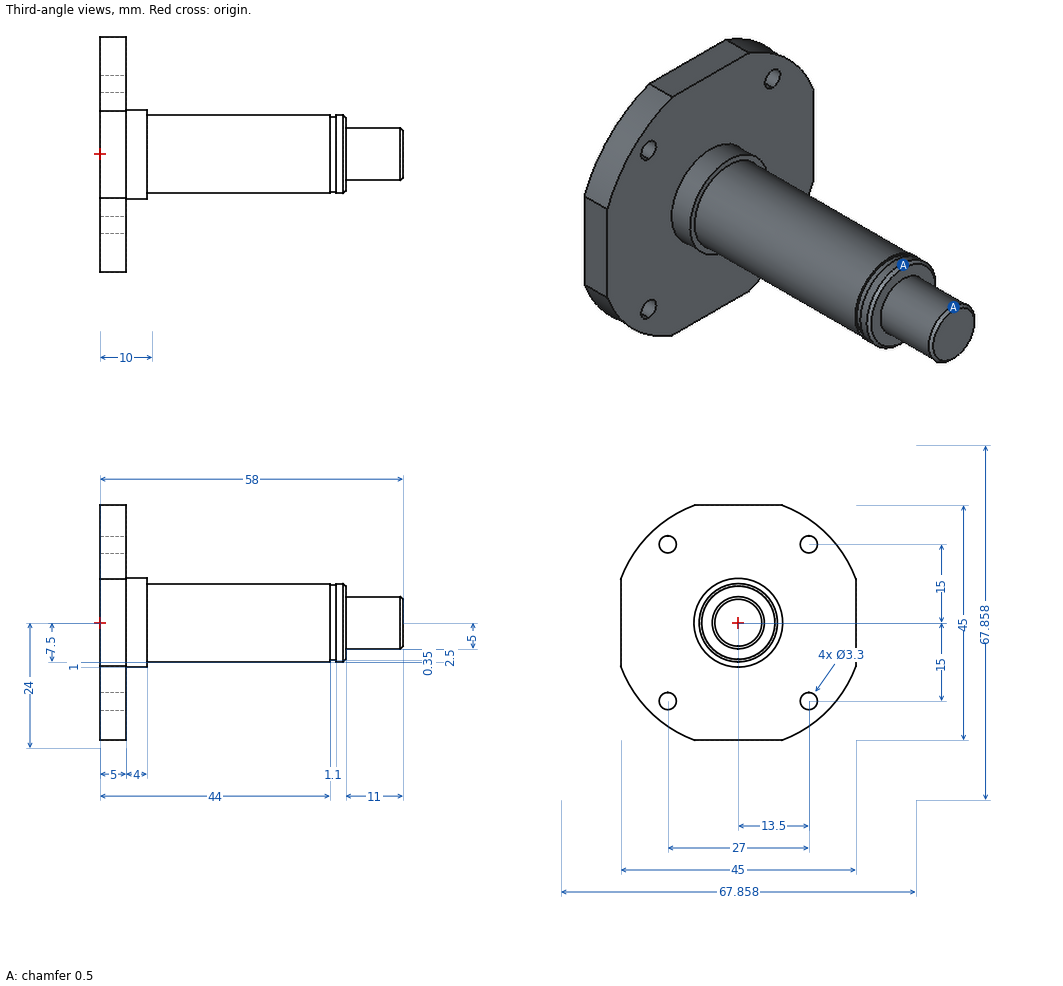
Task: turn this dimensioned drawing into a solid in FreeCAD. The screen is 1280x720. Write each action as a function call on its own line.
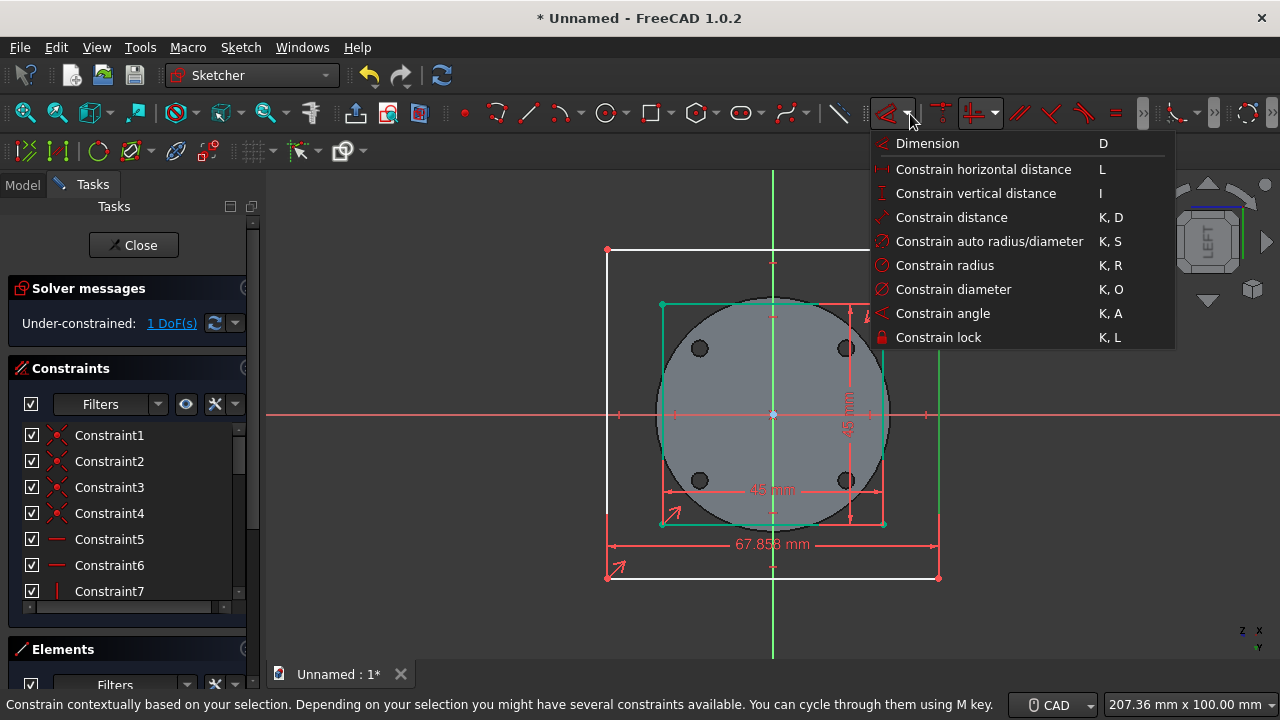
click(1023, 193)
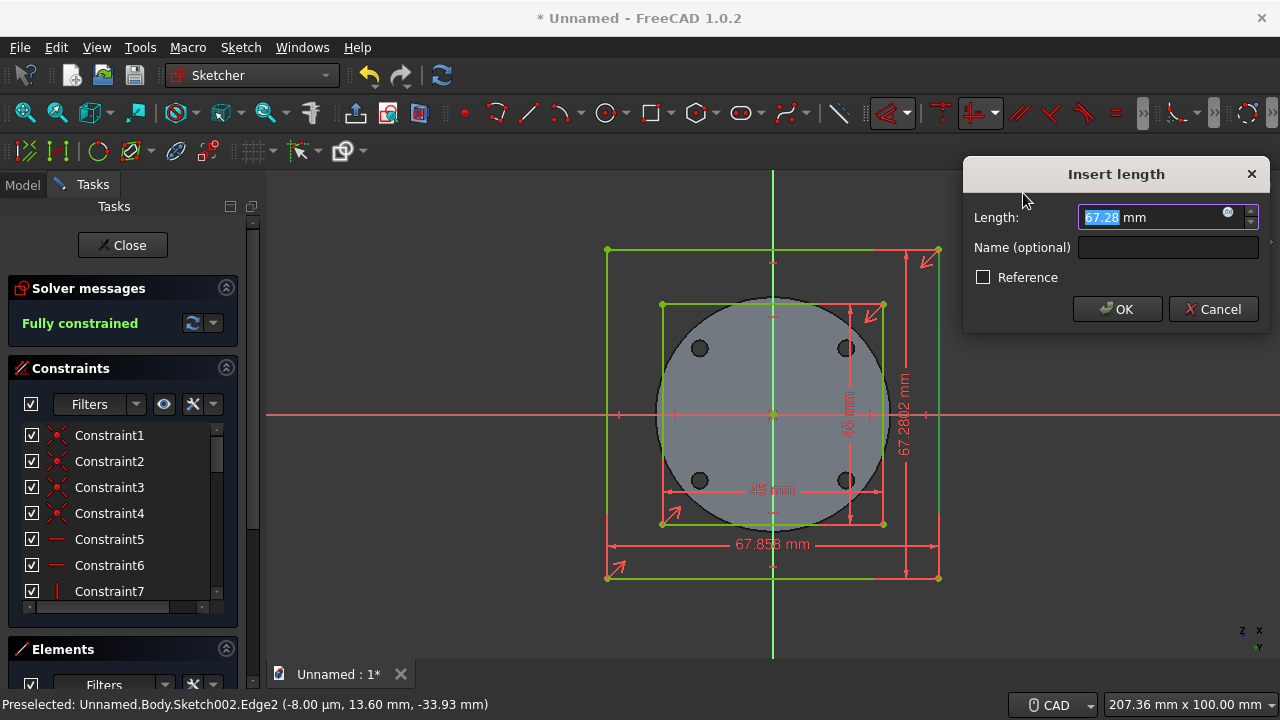
text(67.858)
key(Return)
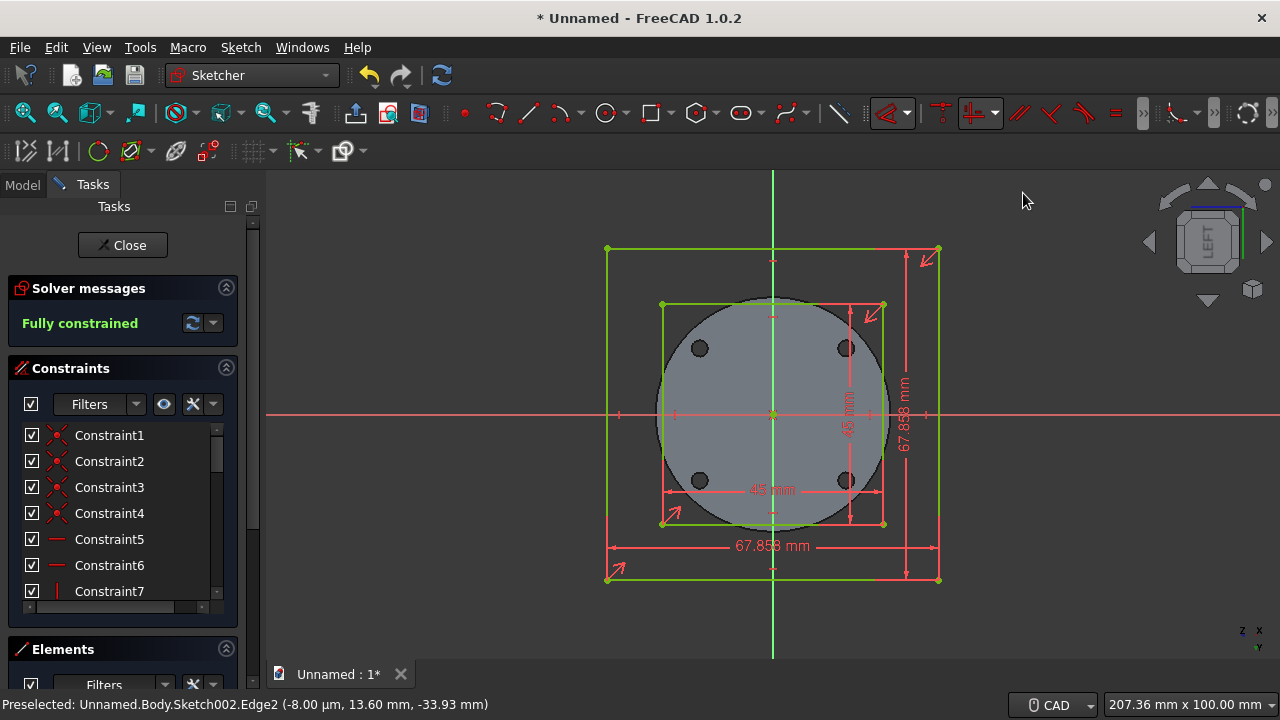
click(123, 245)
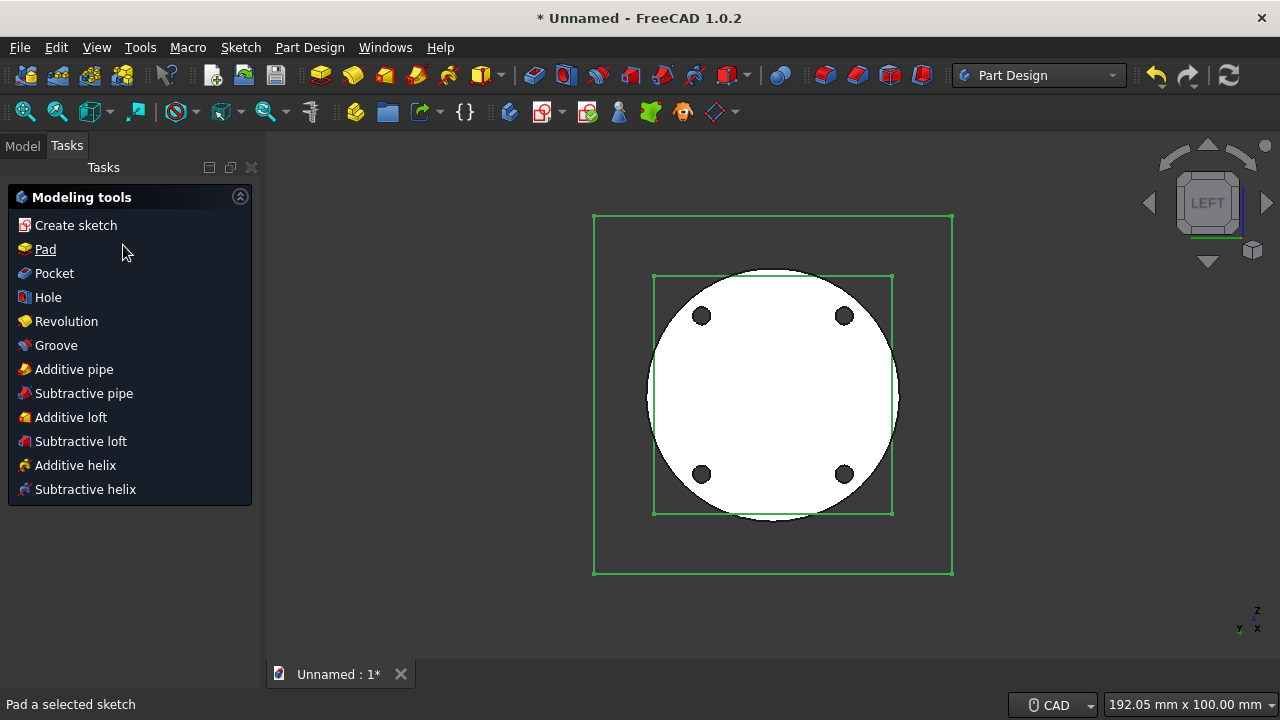
click(536, 76)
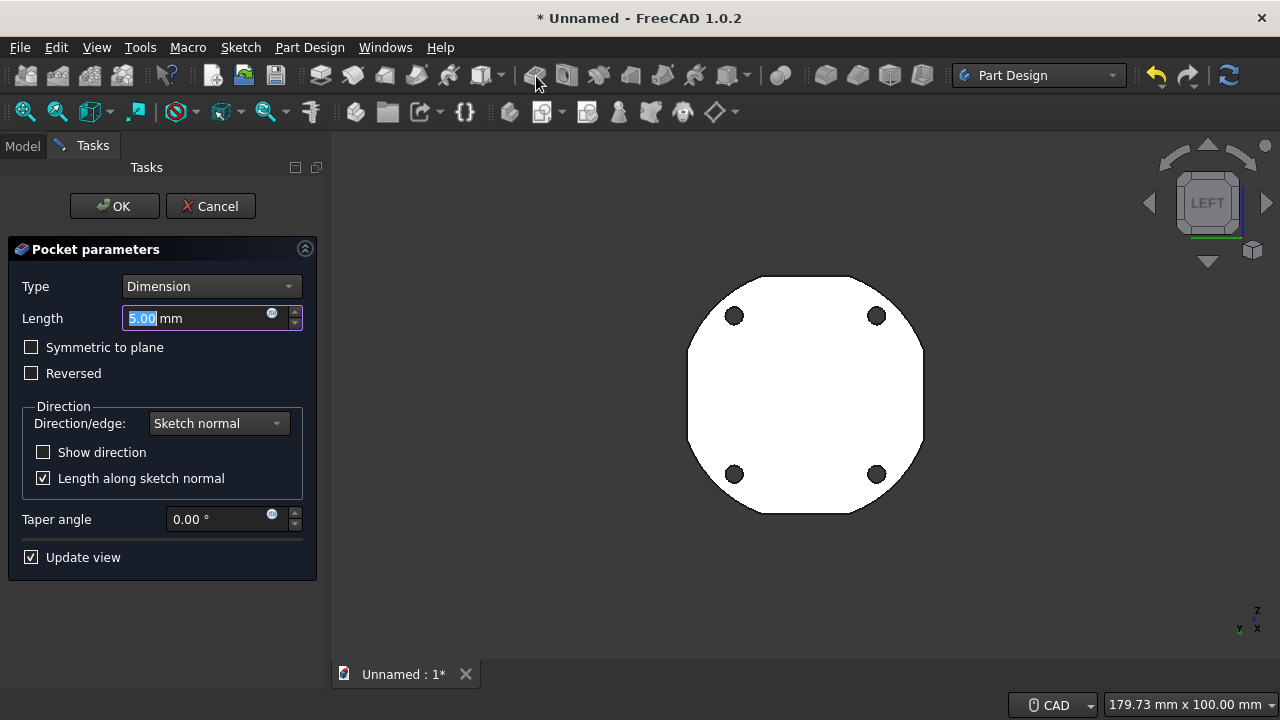
text(10)
key(Tab)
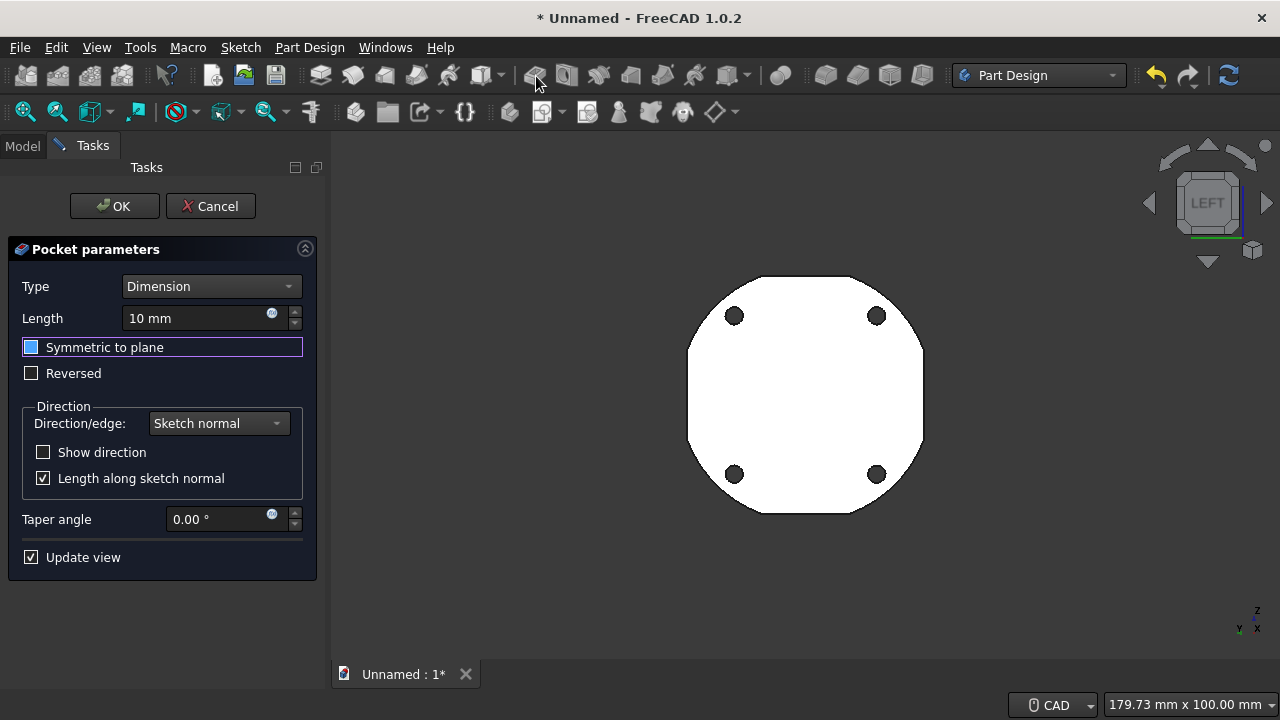
click(115, 206)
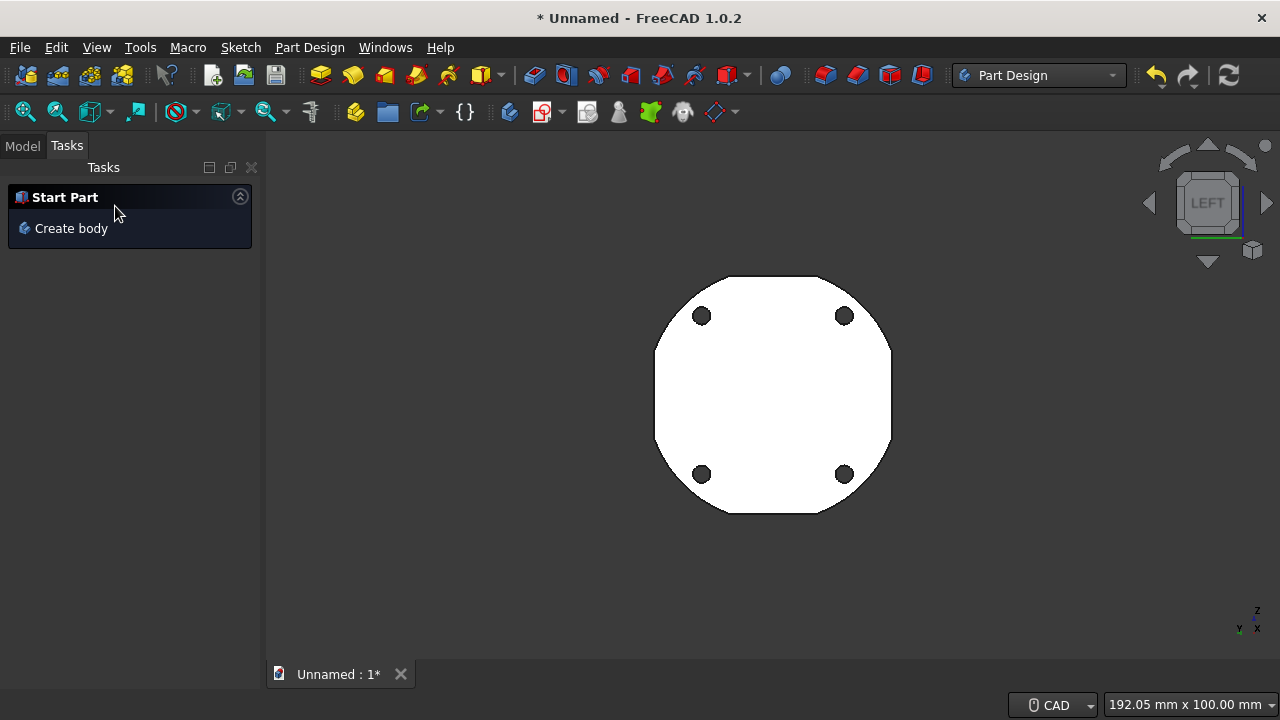
key(0)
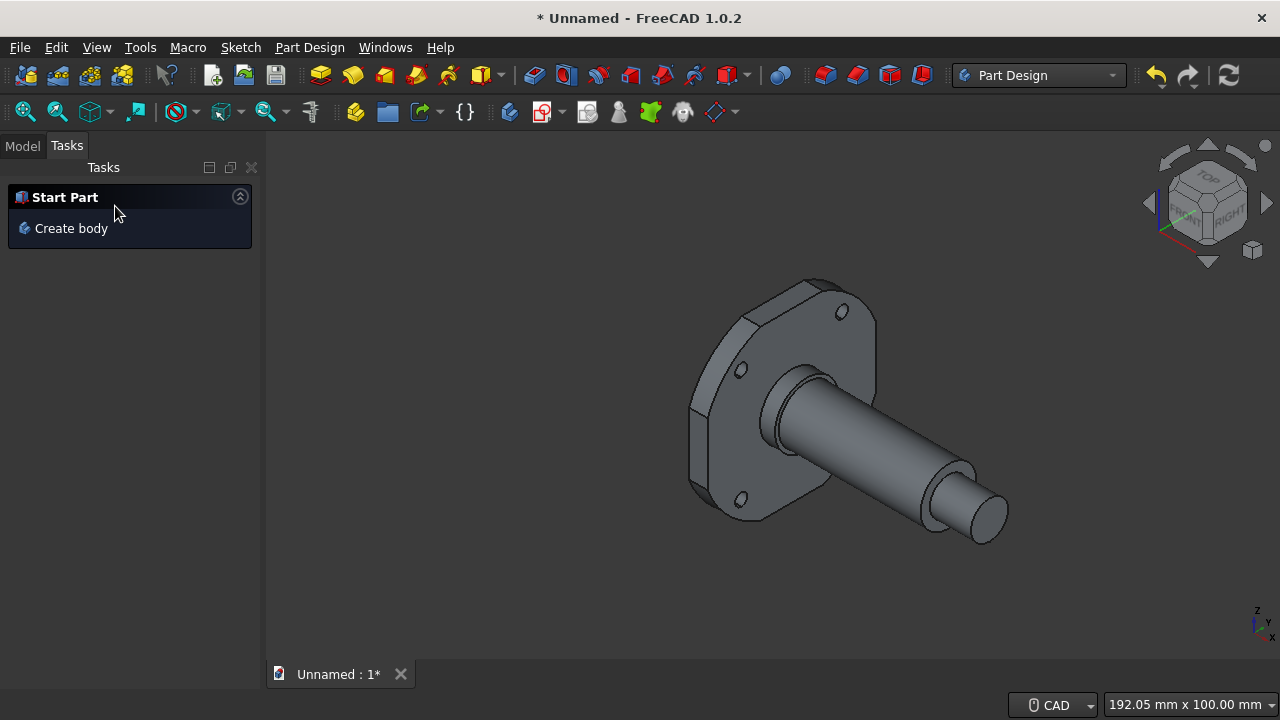
click(26, 112)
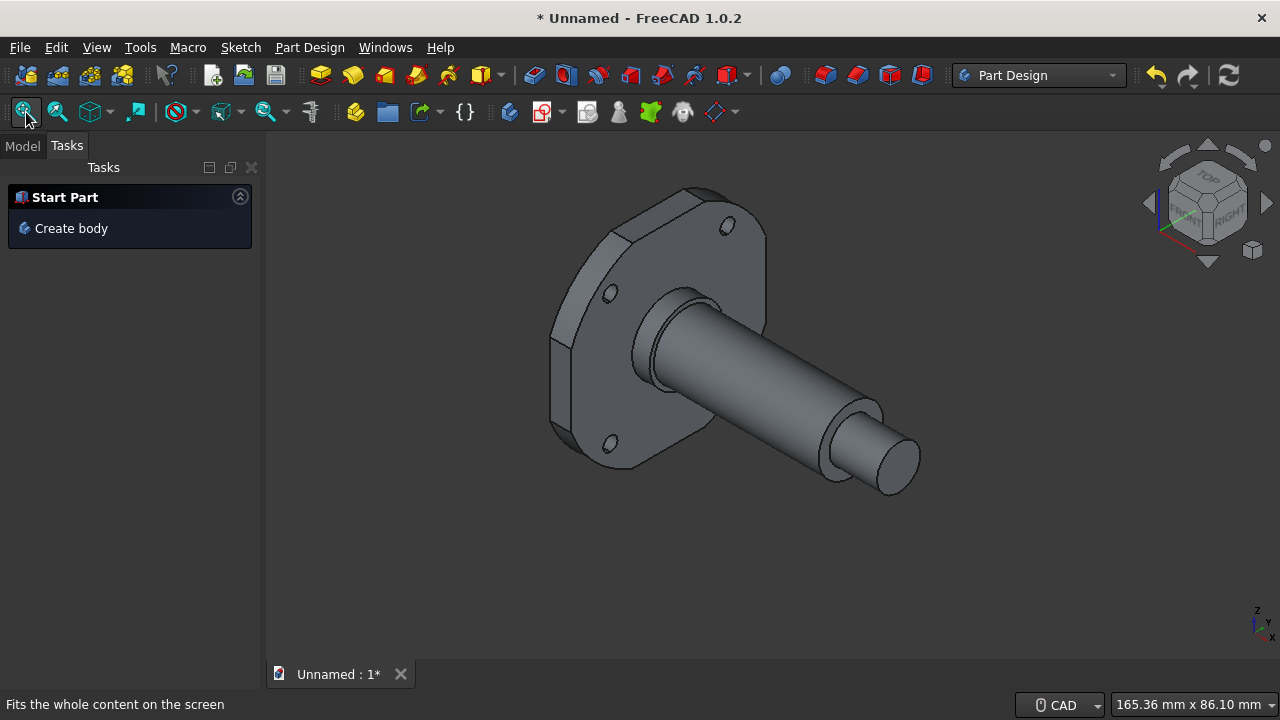
click(899, 442)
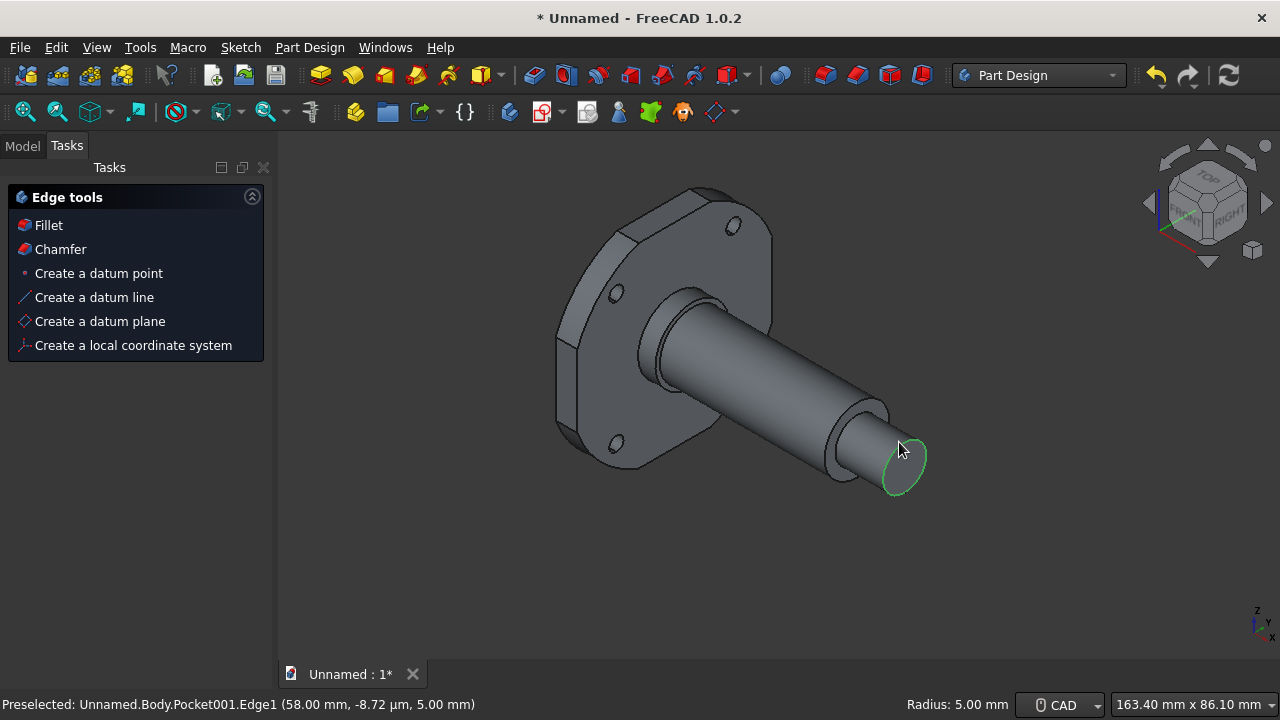
click(857, 402, ctrl)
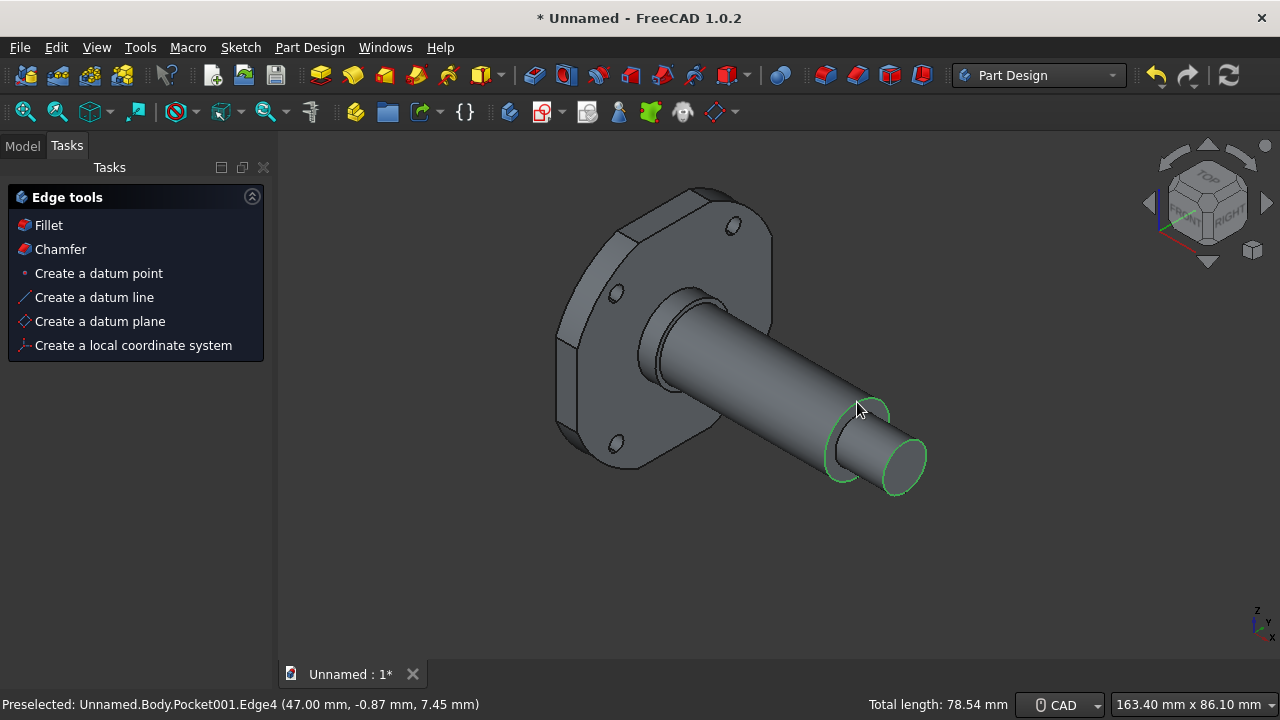
click(858, 76)